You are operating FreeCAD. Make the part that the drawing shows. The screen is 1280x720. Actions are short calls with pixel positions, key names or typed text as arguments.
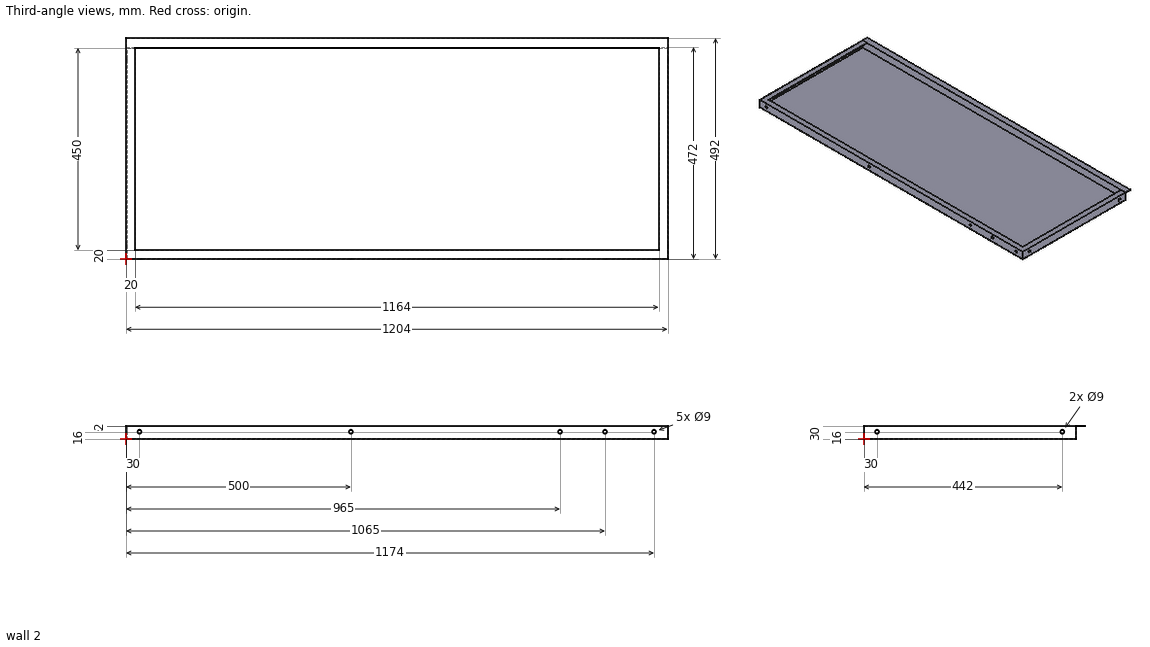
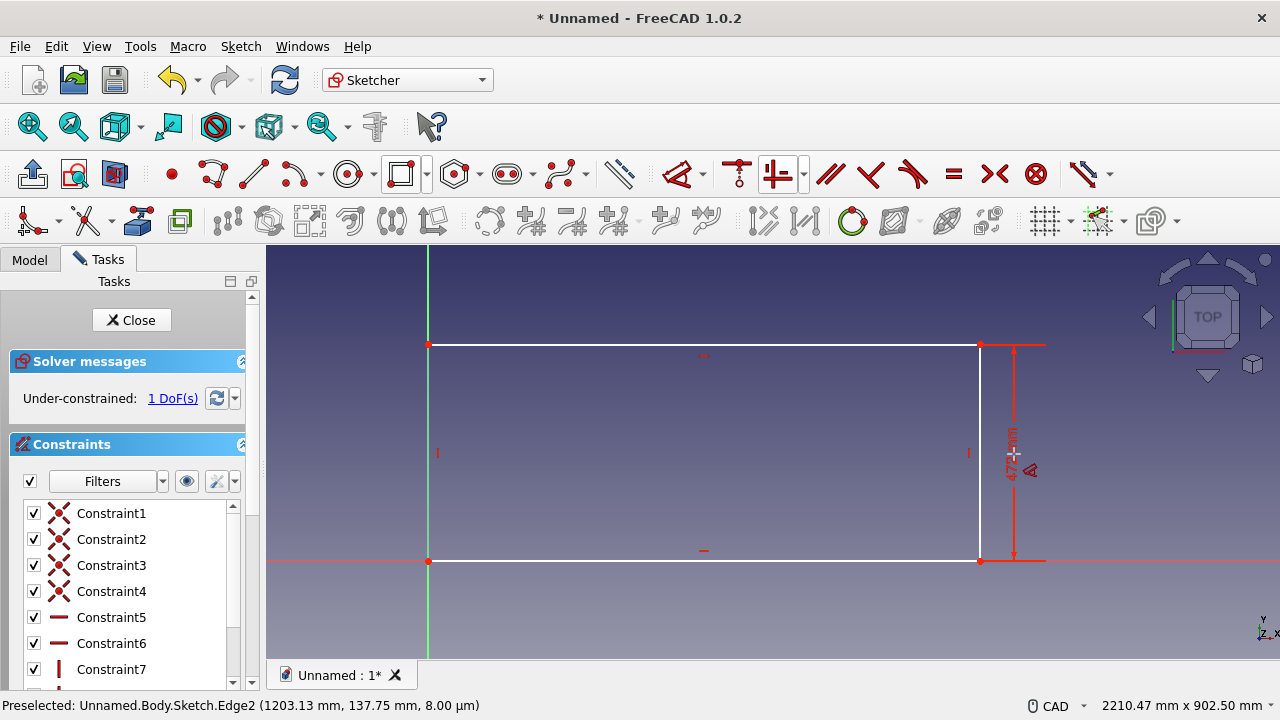
click(594, 561)
click(704, 595)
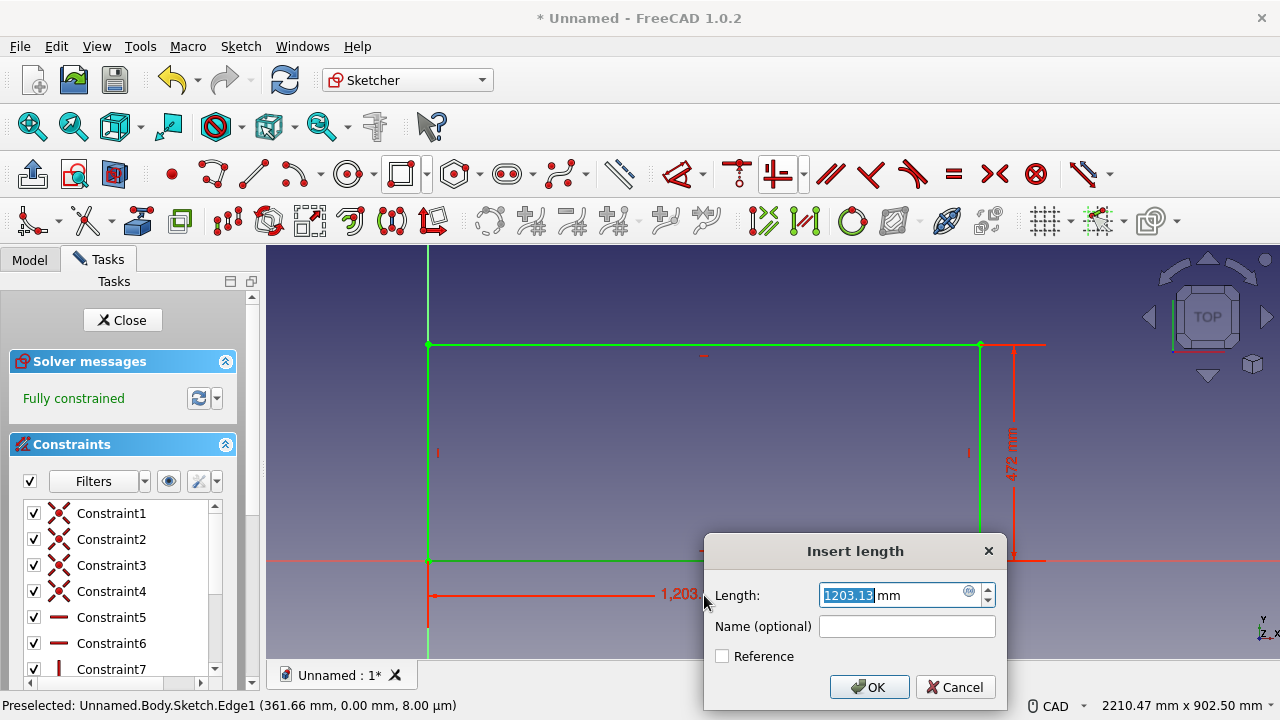
text(1204)
key(Return)
key(Escape)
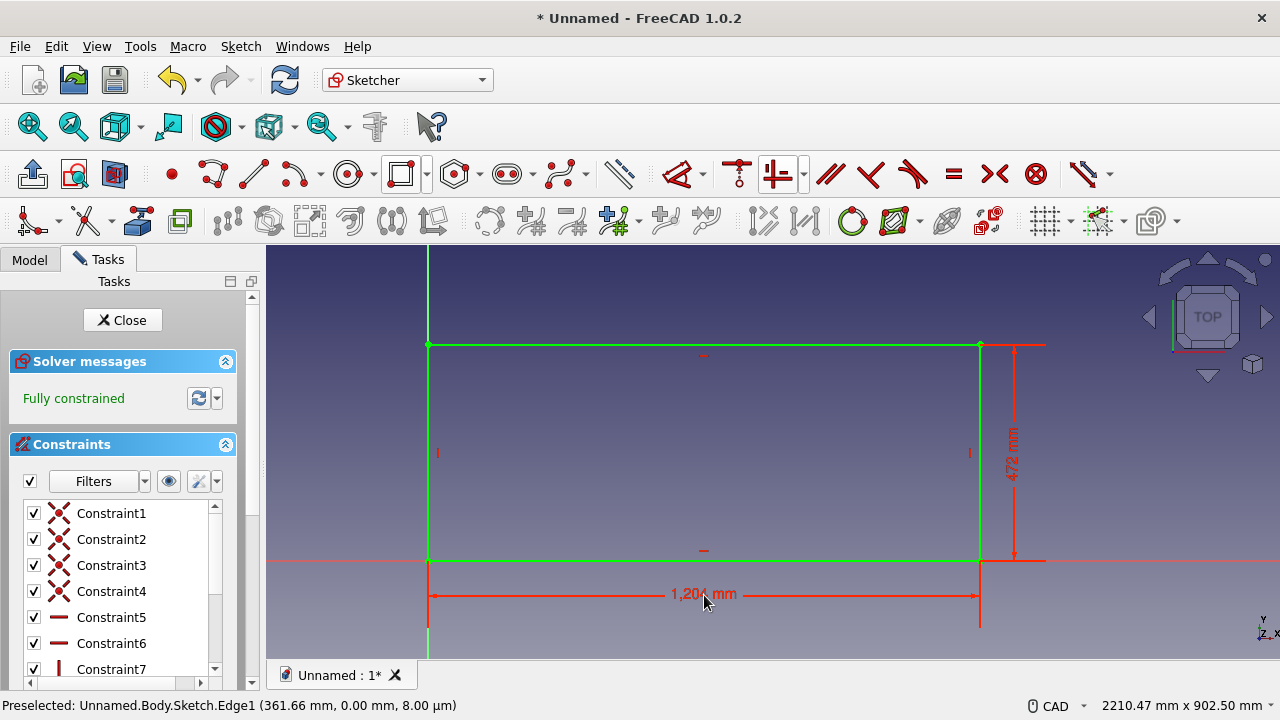
click(123, 320)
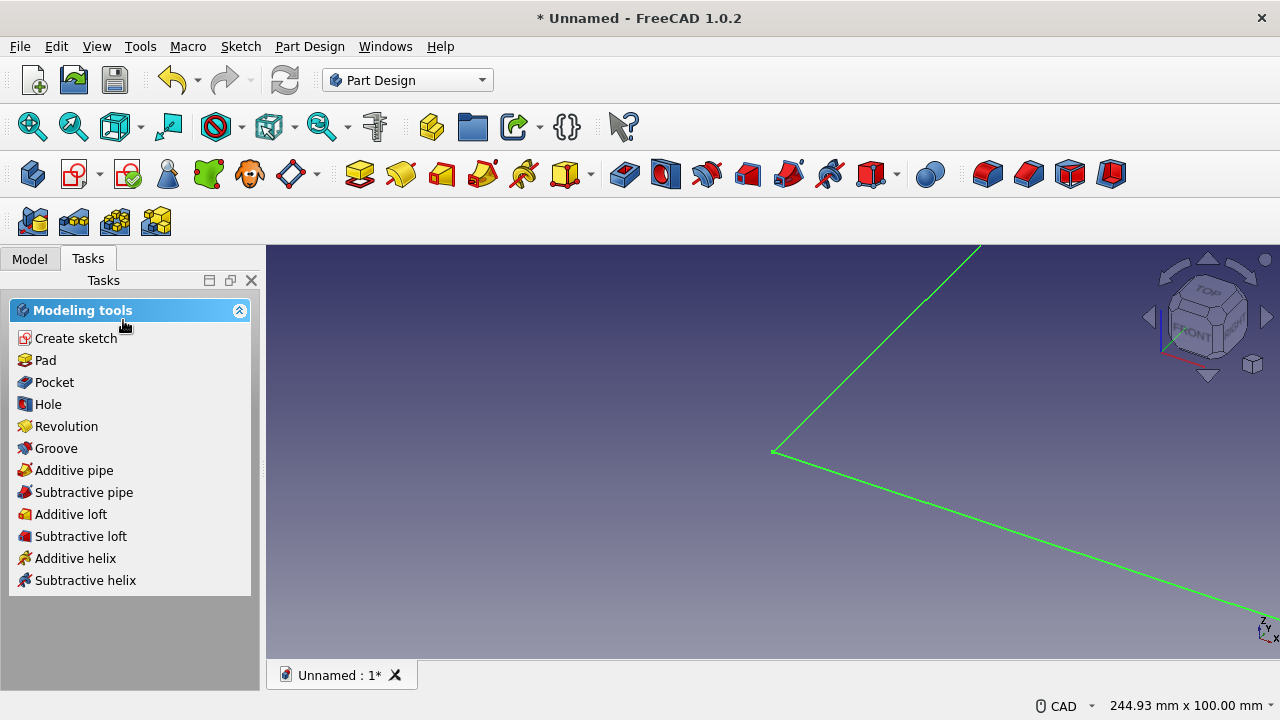
click(360, 174)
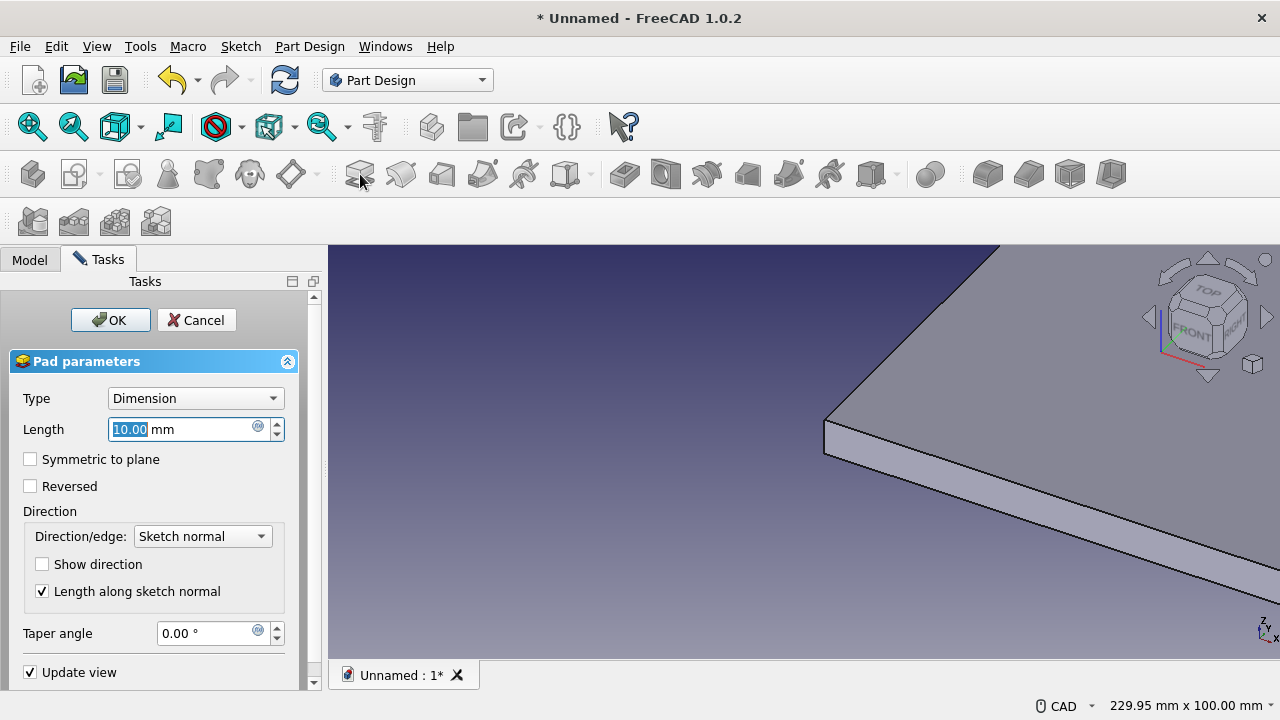
text(30)
key(Tab)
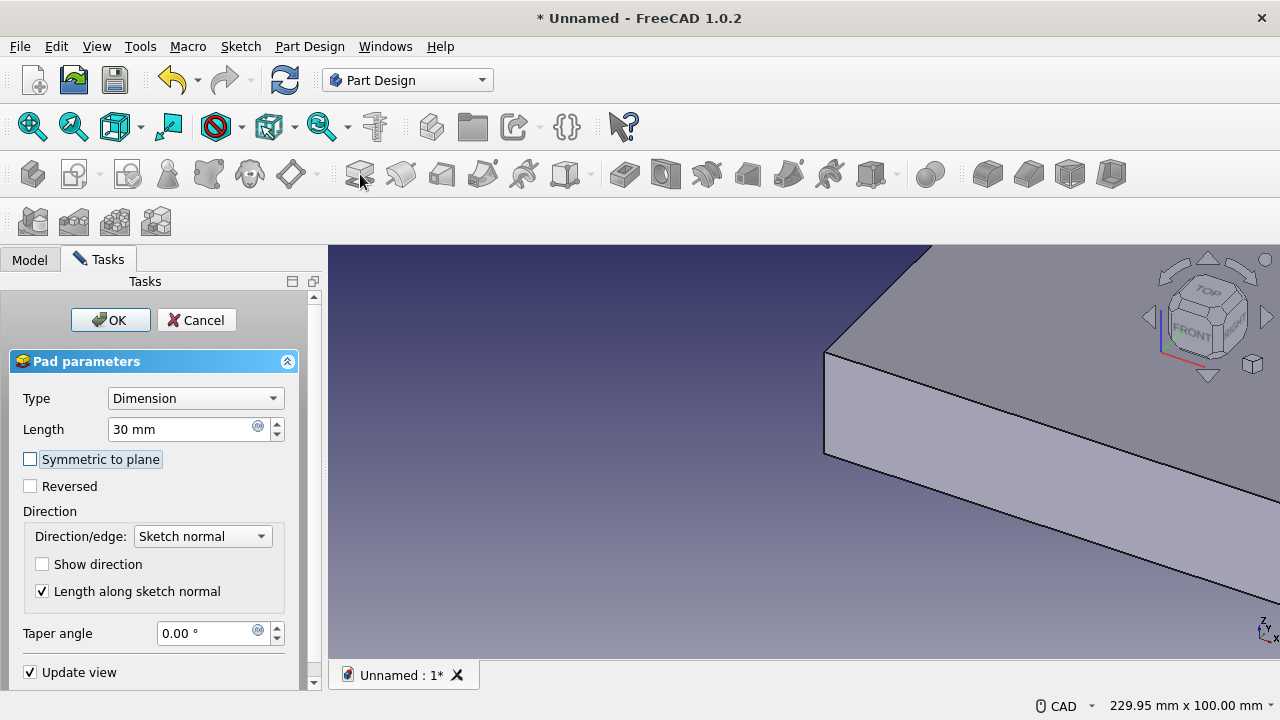
click(111, 320)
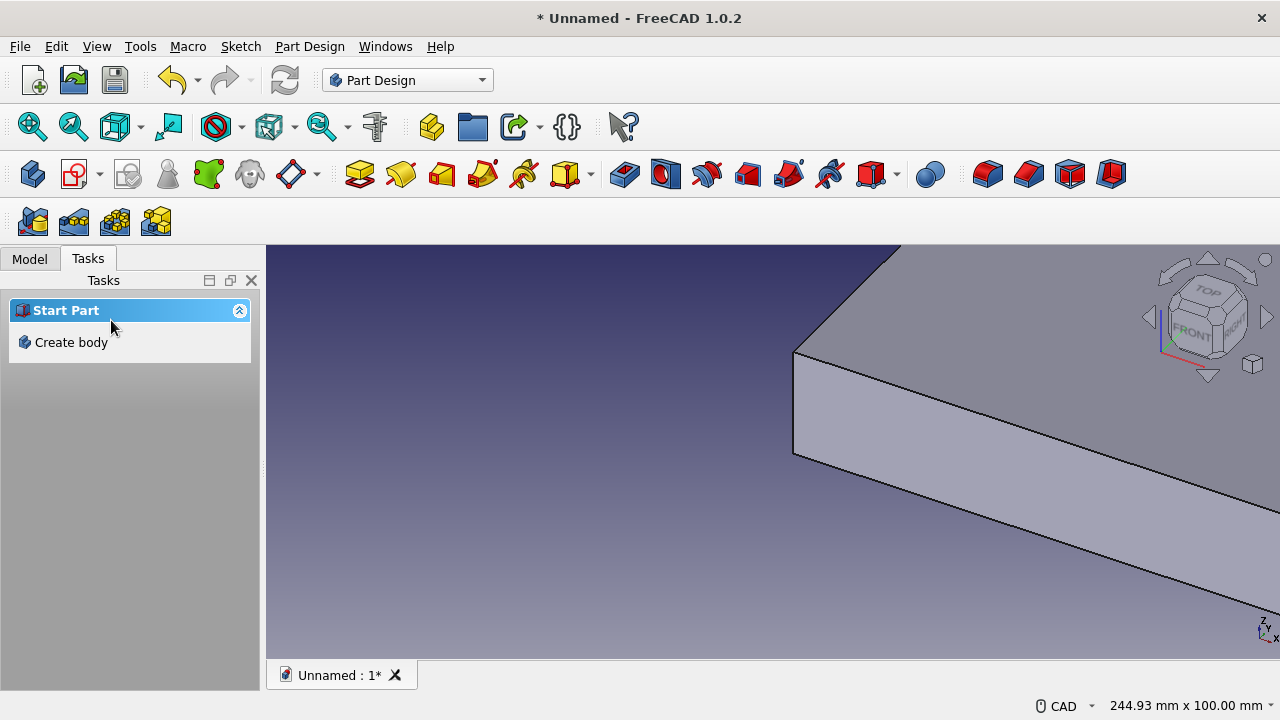
key(v)
key(f)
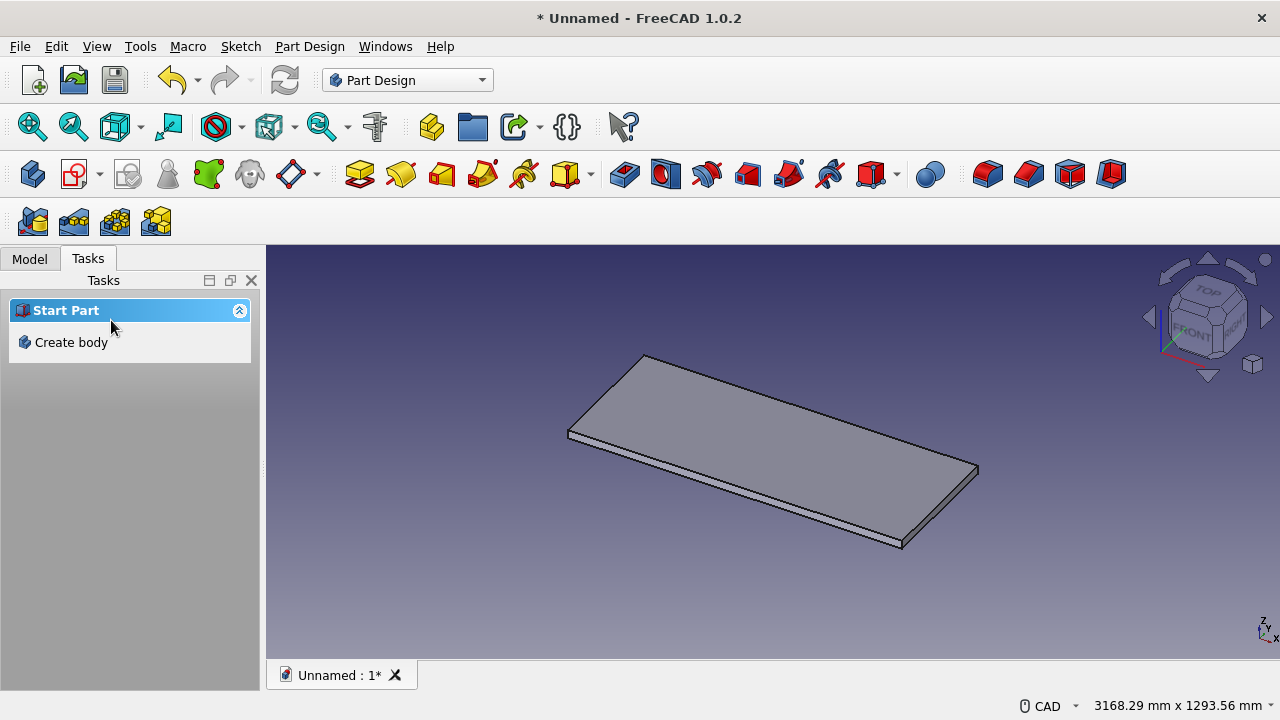
click(868, 479)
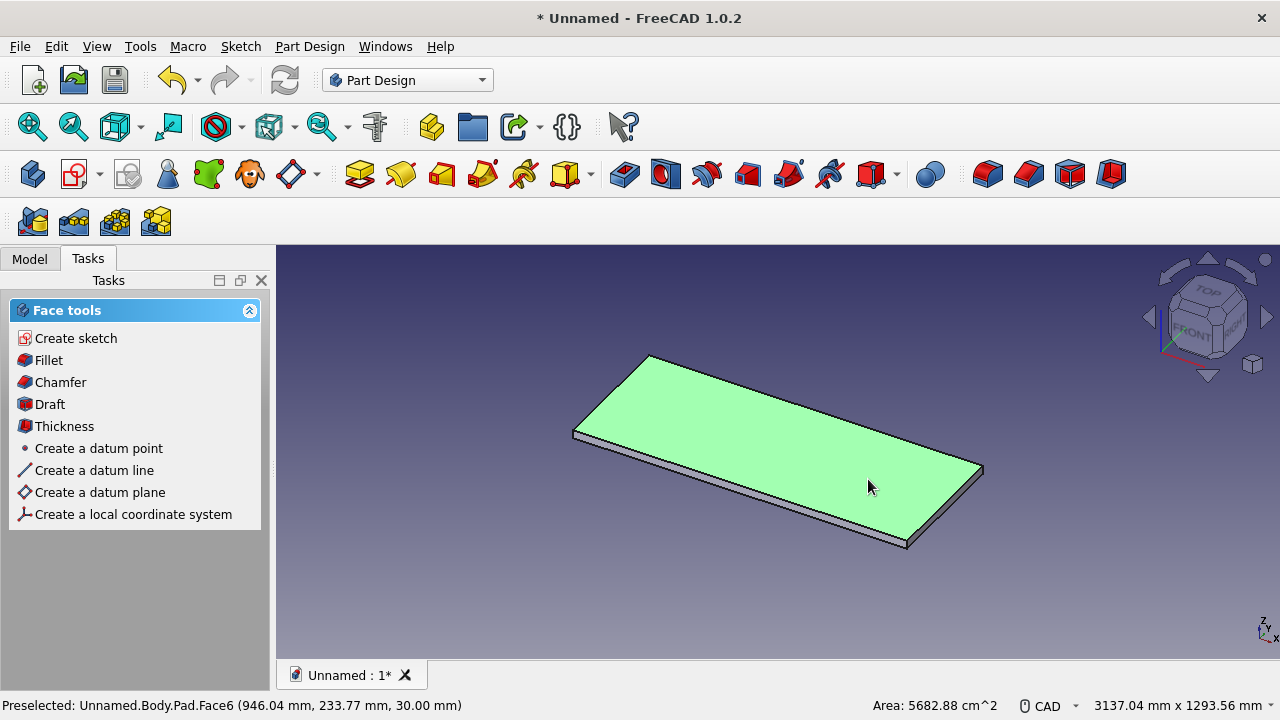
click(1111, 174)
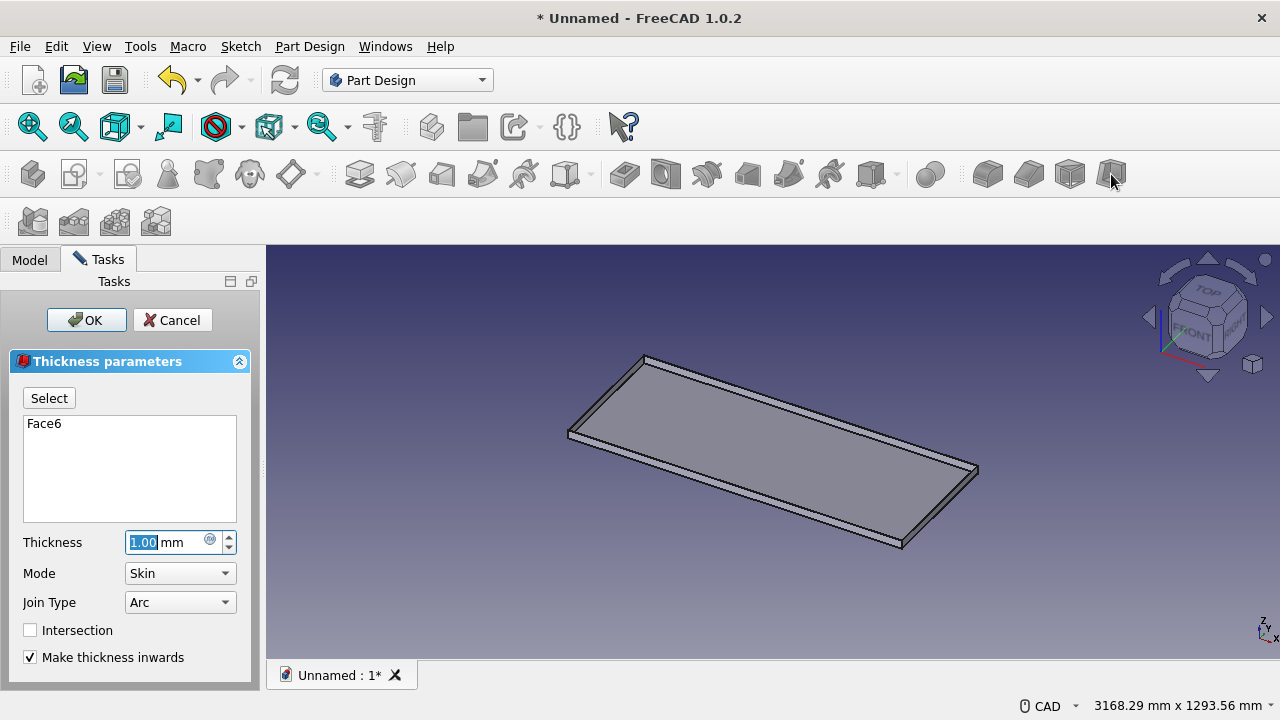
text(2)
key(Tab)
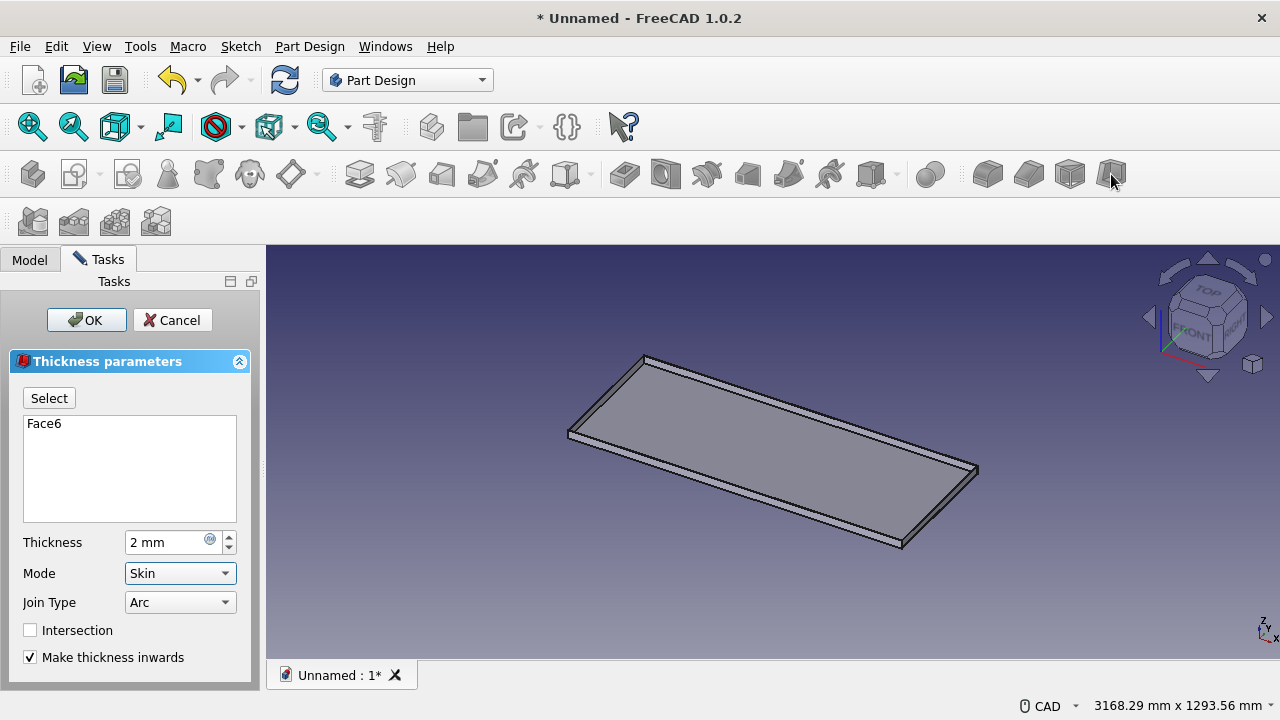
click(181, 602)